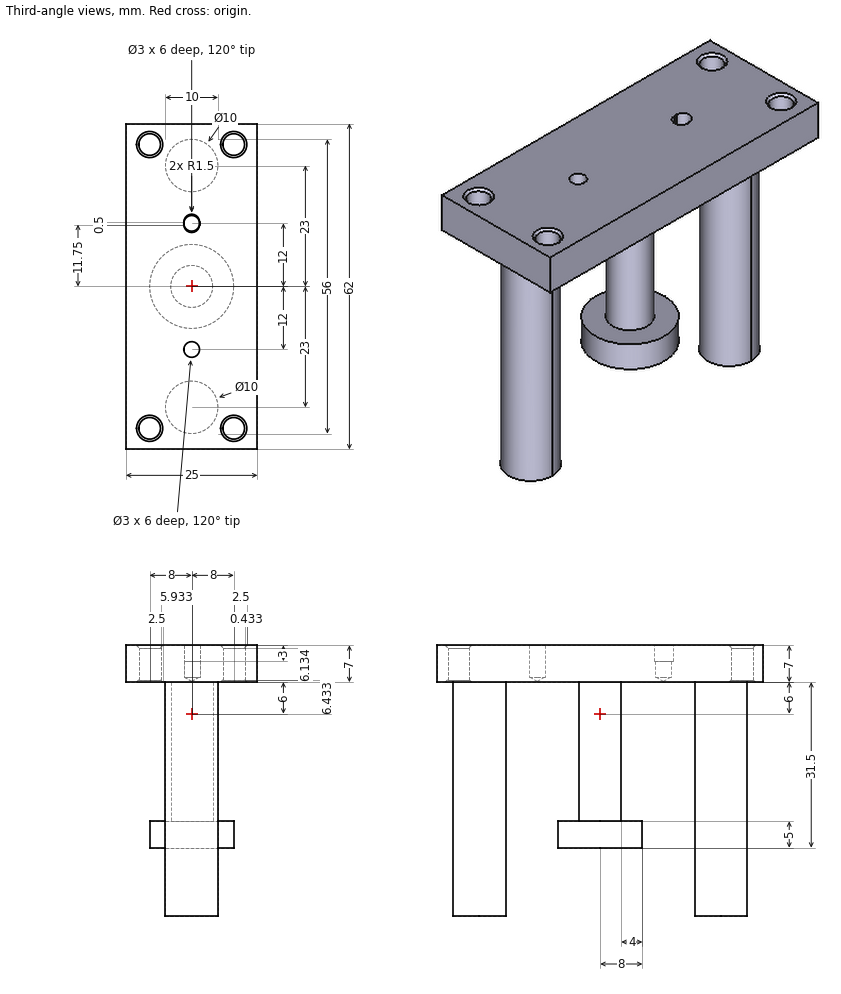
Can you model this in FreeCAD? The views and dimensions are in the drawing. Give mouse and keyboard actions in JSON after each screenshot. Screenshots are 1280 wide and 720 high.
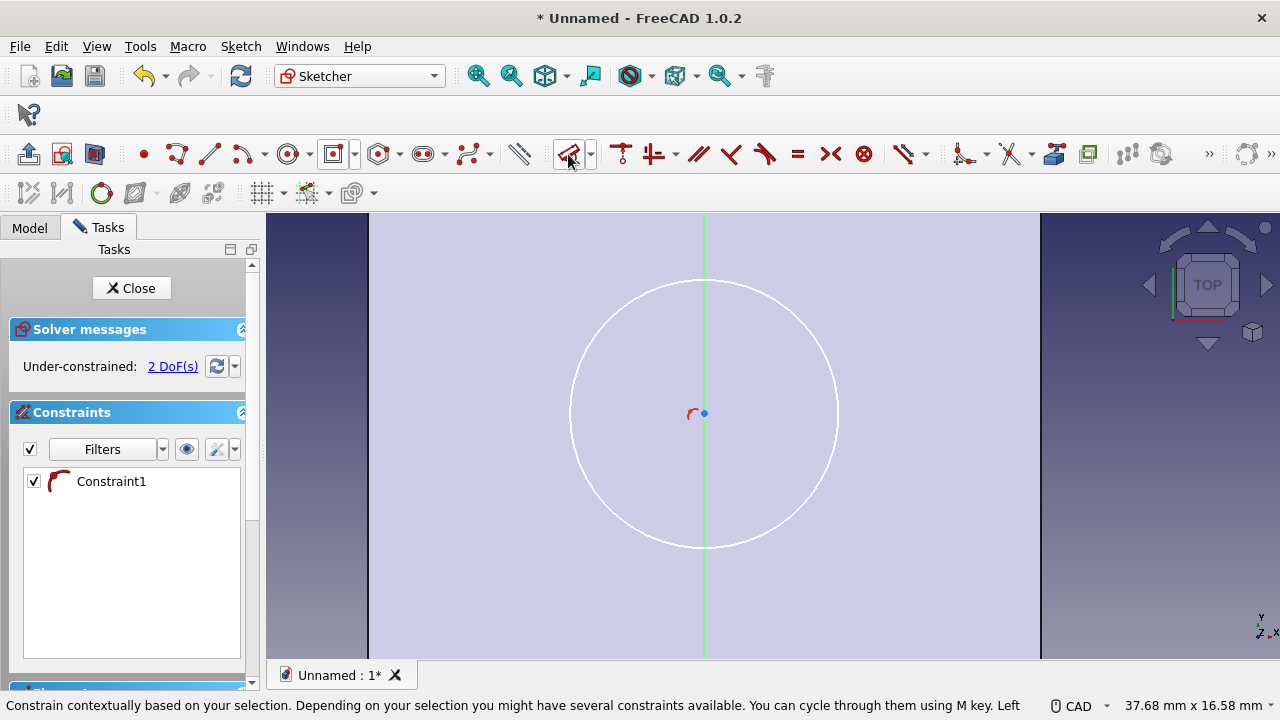
{"action": "left_click", "coordinate": [799, 319]}
{"action": "left_click", "coordinate": [822, 296]}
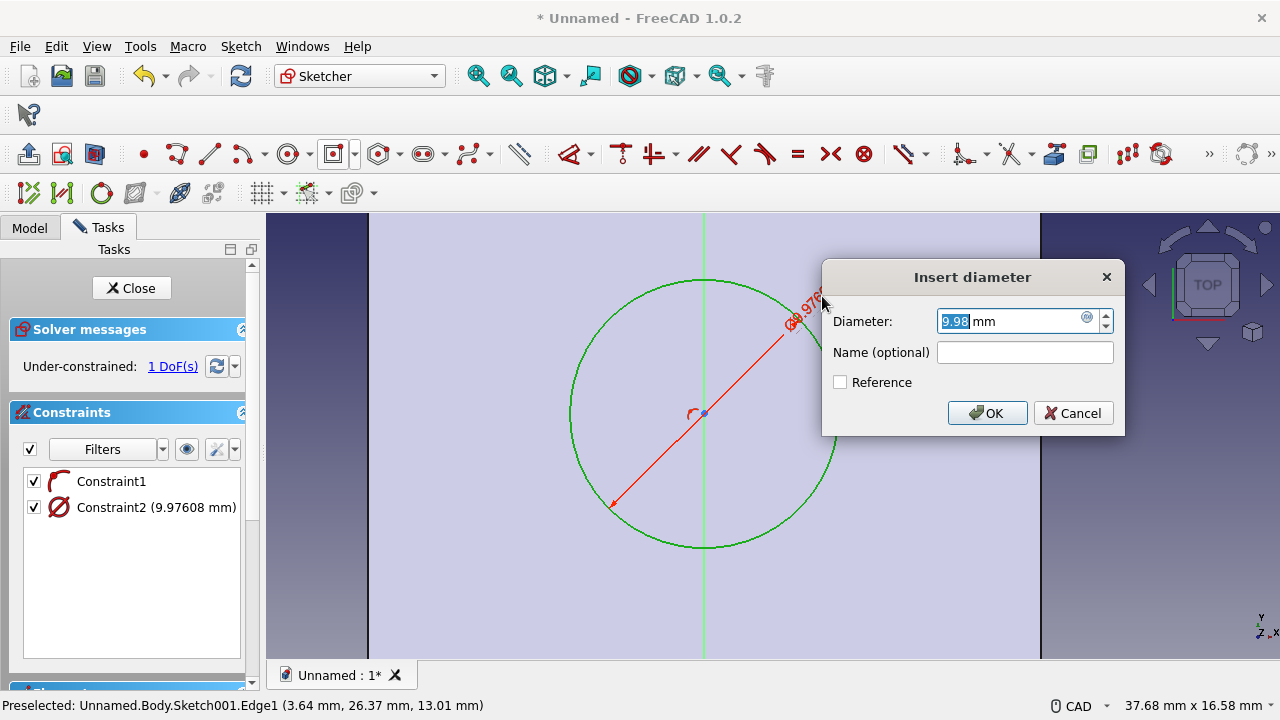
{"action": "type", "text": "10"}
{"action": "key", "text": "Return"}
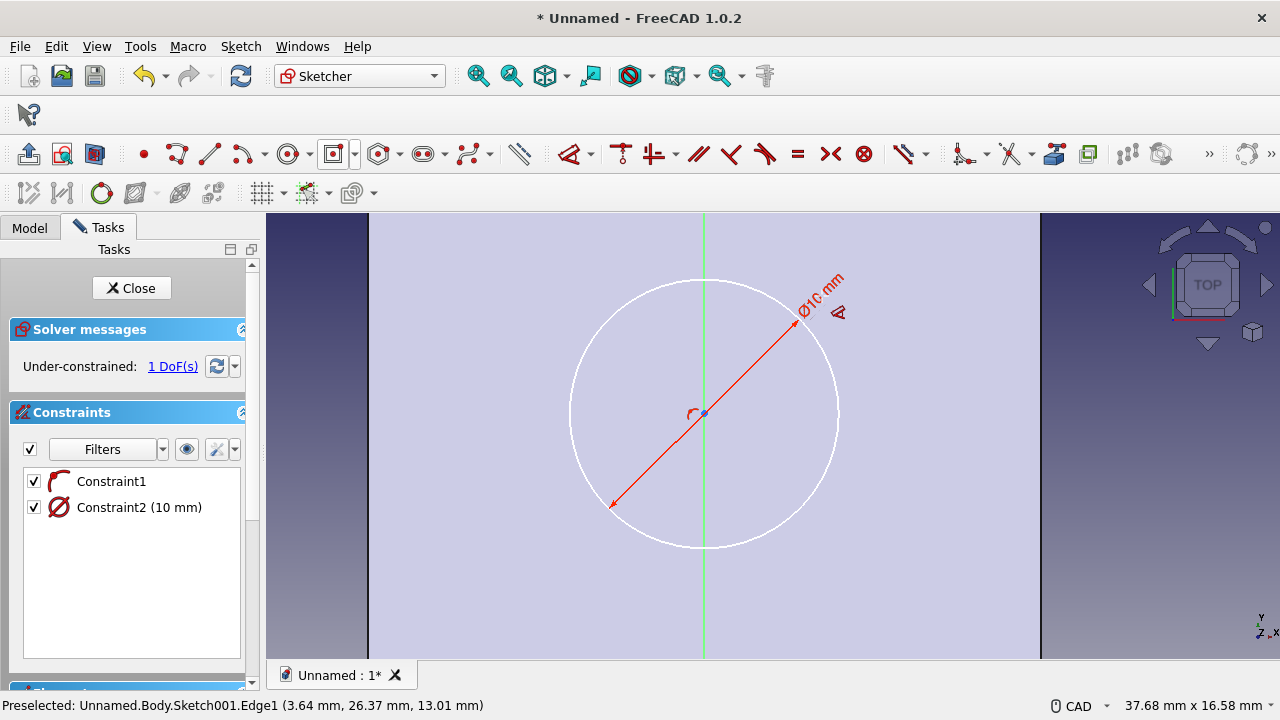
{"action": "left_click", "coordinate": [704, 414]}
{"action": "left_click", "coordinate": [738, 522]}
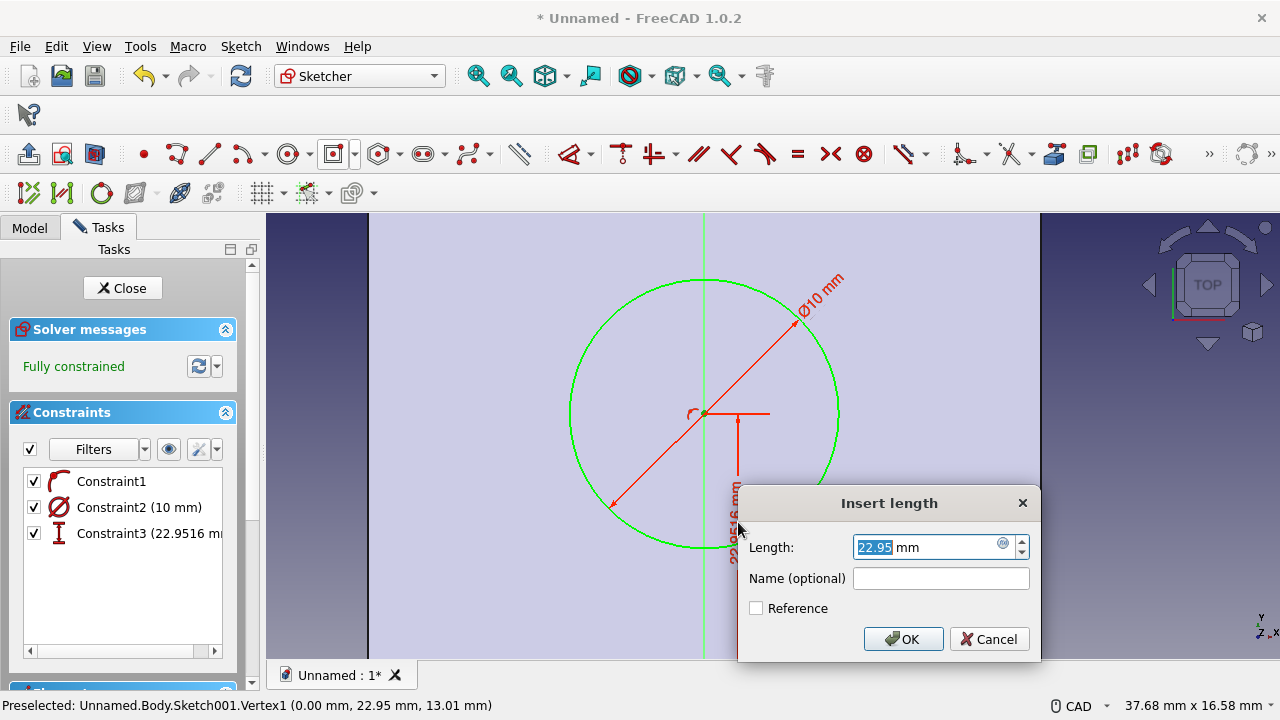
{"action": "type", "text": "23"}
{"action": "key", "text": "Return"}
{"action": "key", "text": "Escape"}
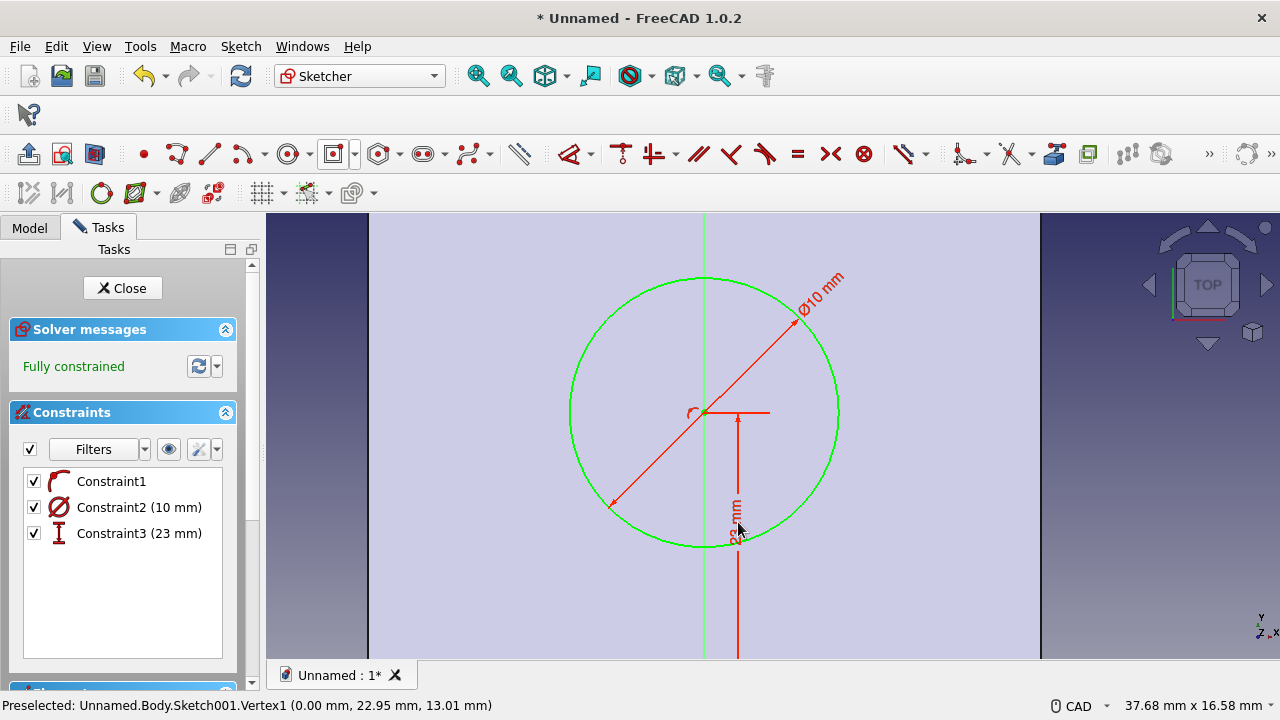
{"action": "left_click", "coordinate": [123, 288]}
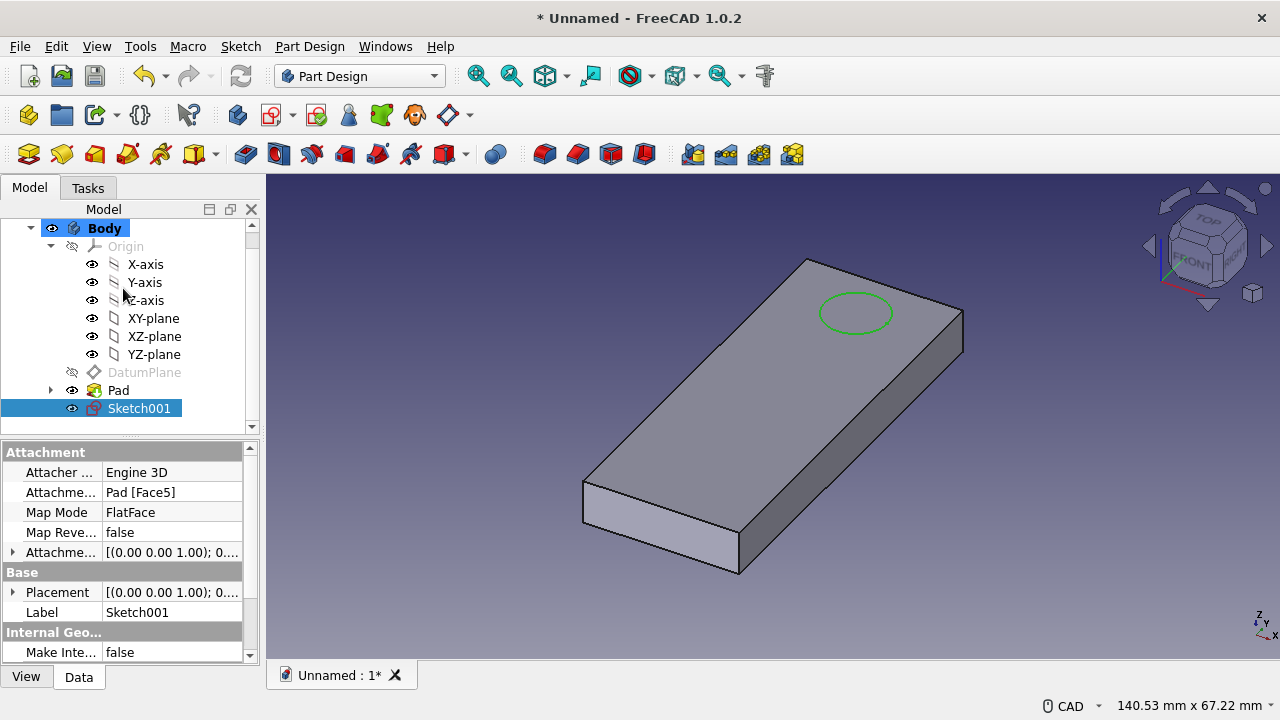
{"action": "left_click", "coordinate": [29, 154]}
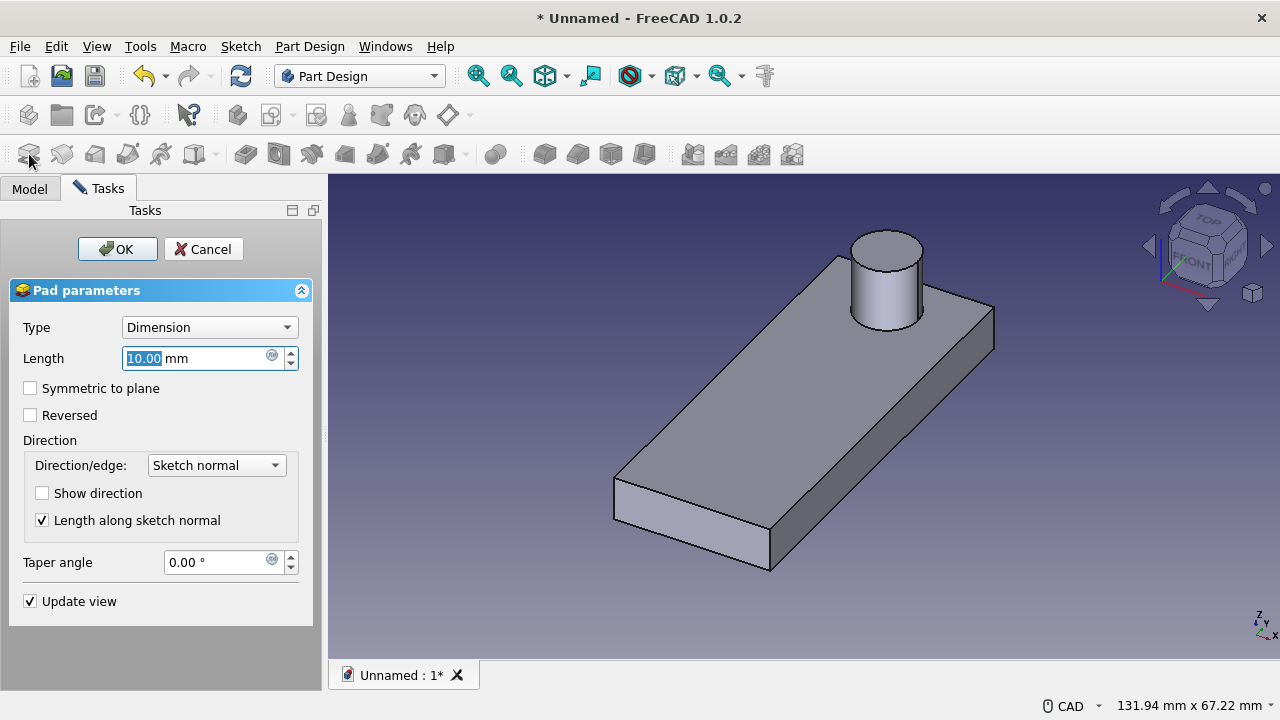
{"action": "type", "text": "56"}
{"action": "key", "text": "Tab"}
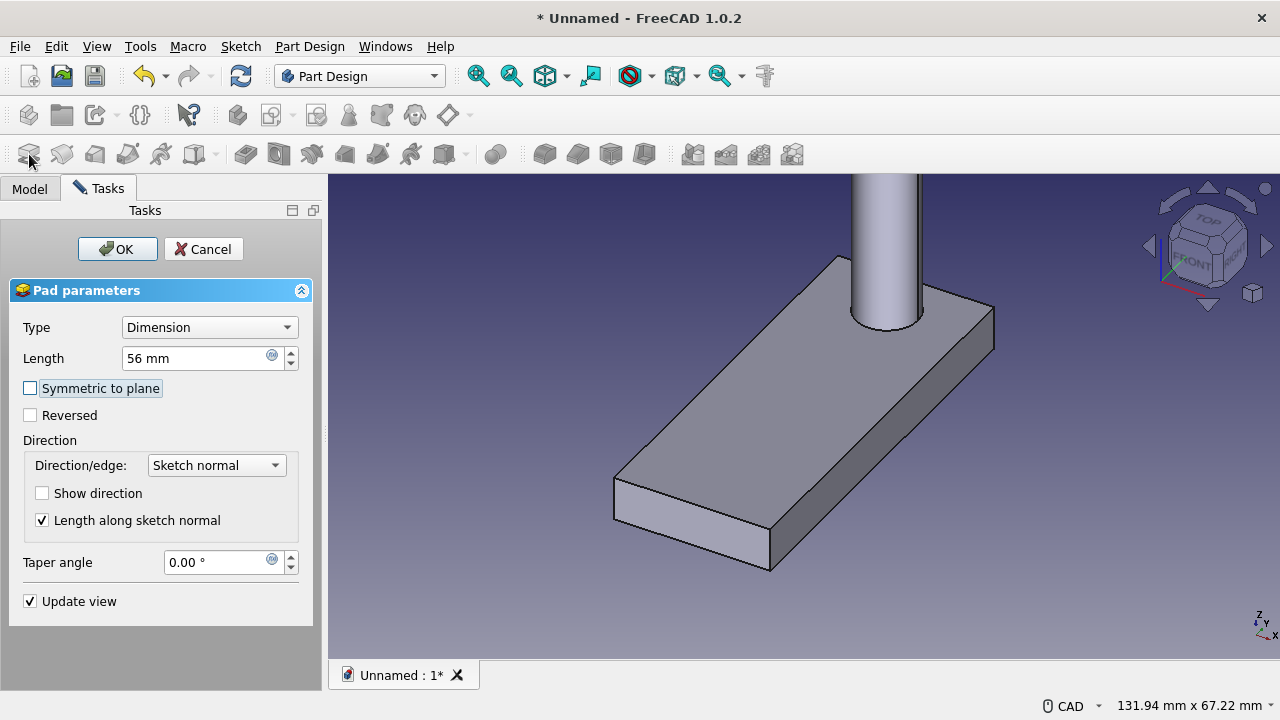
{"action": "left_click", "coordinate": [31, 415]}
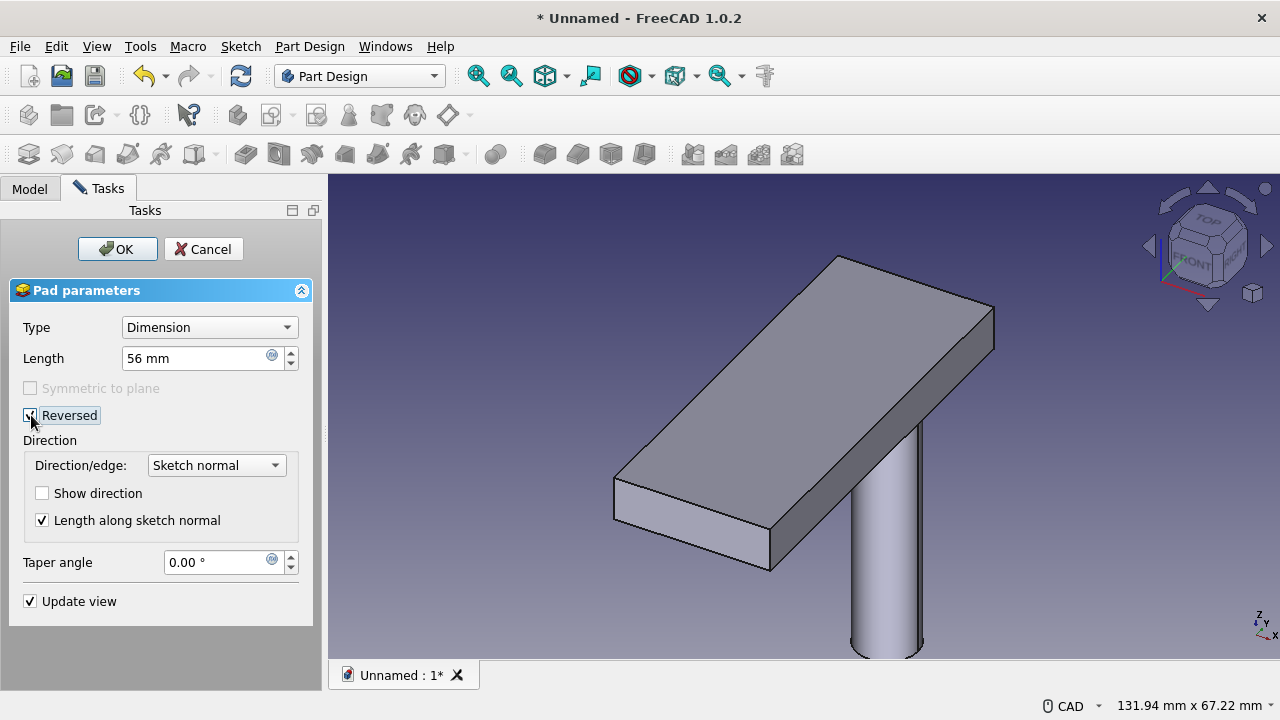
{"action": "left_click", "coordinate": [118, 249]}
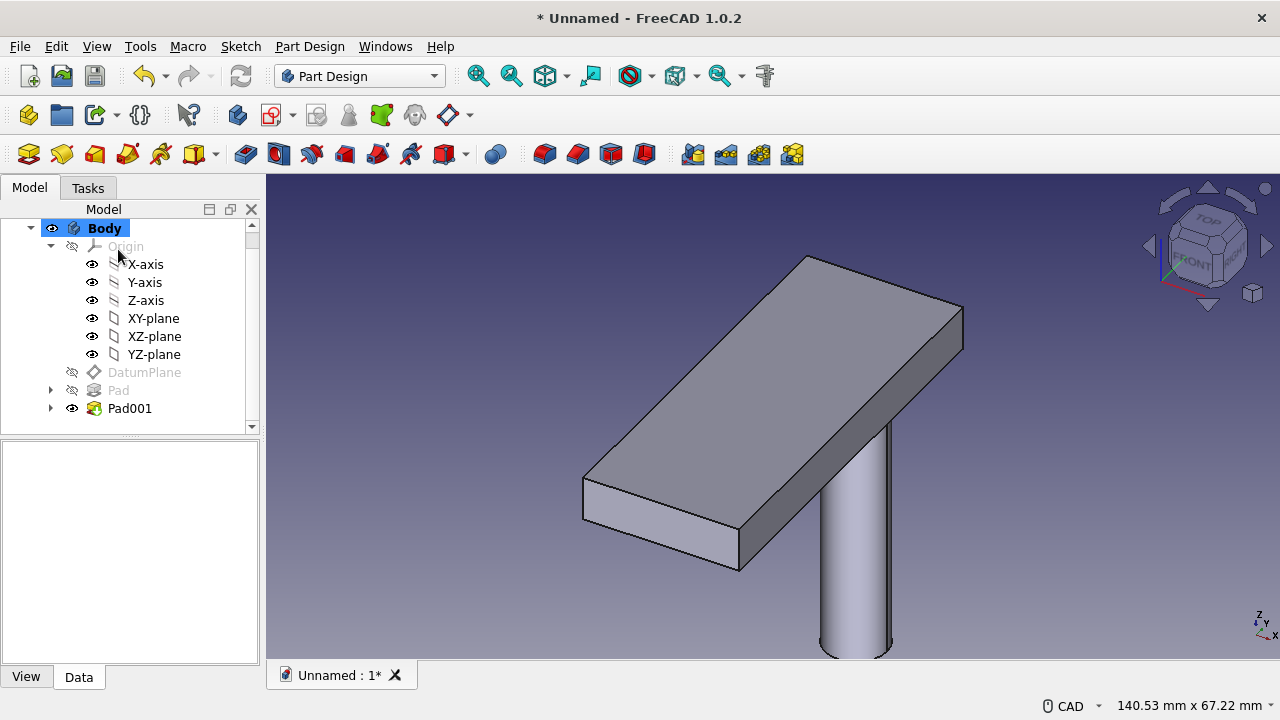
{"action": "left_click", "coordinate": [479, 76]}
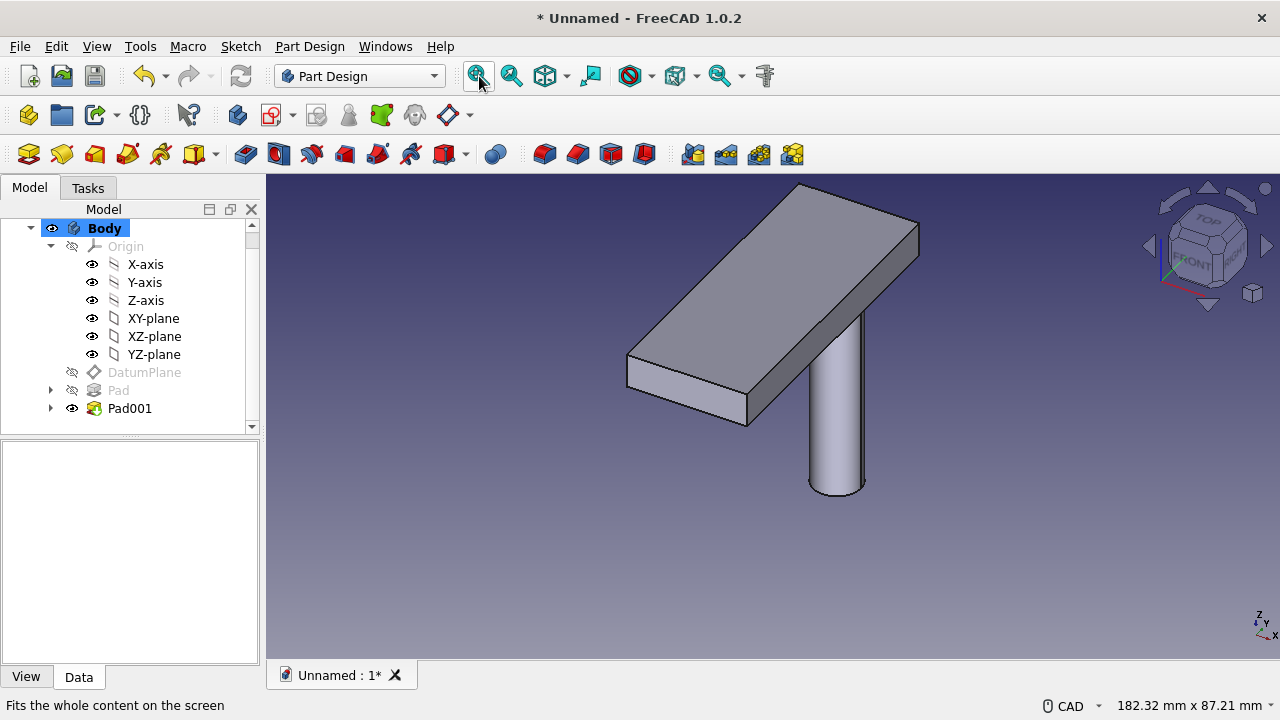
{"action": "left_click", "coordinate": [822, 239]}